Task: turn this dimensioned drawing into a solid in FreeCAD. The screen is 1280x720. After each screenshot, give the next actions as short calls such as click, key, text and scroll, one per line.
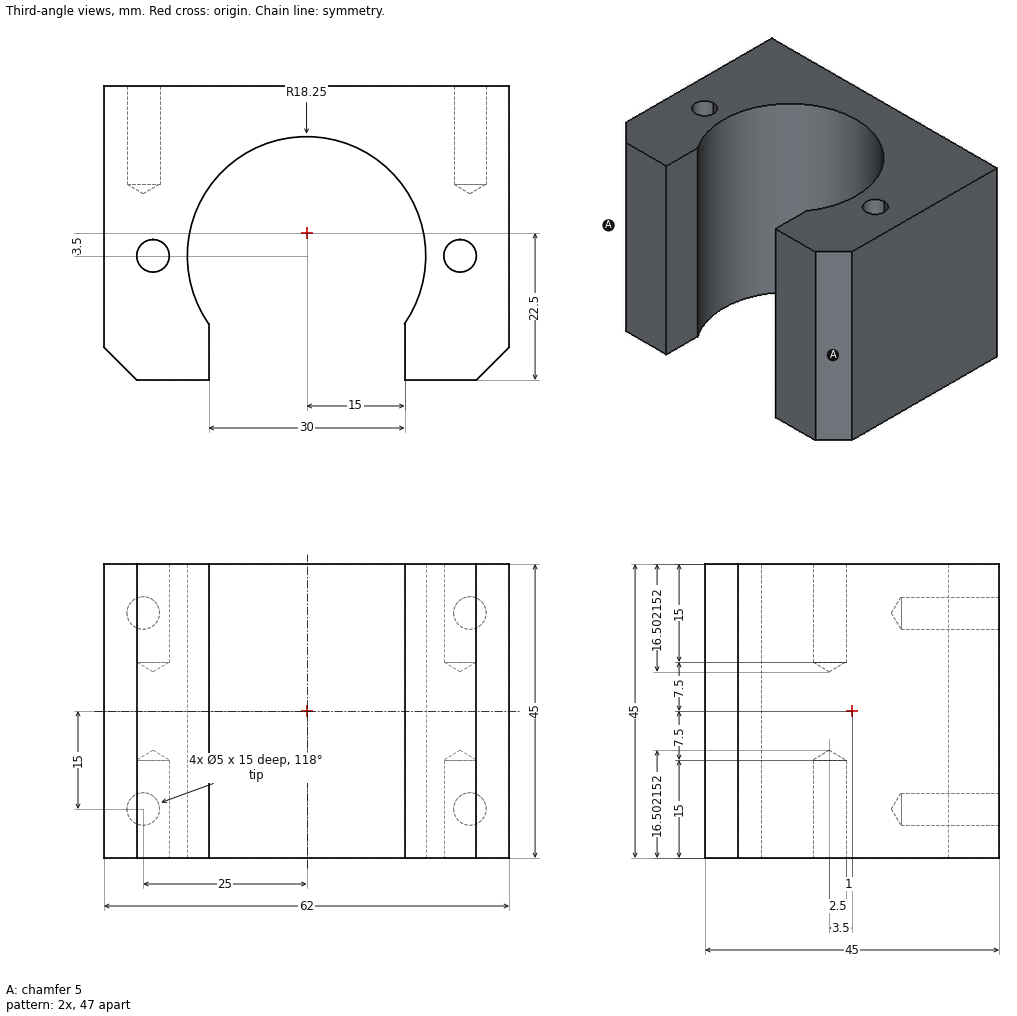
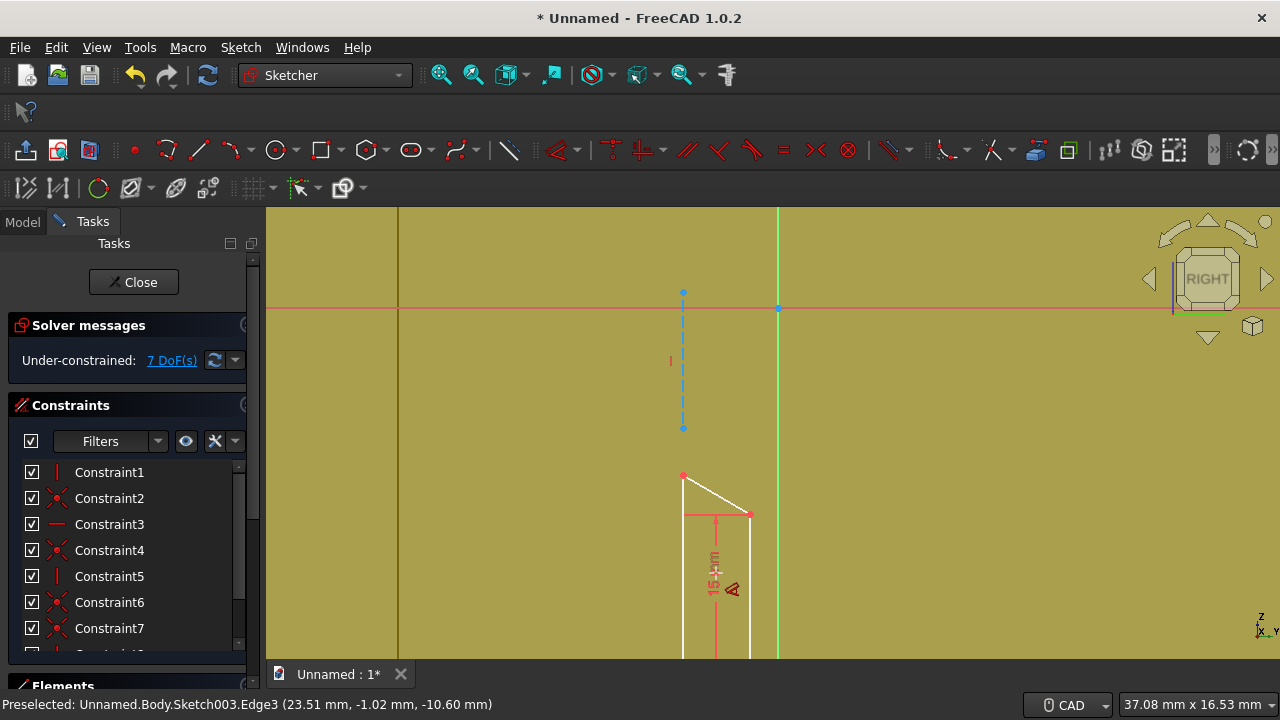
scroll(683, 291, down, 4)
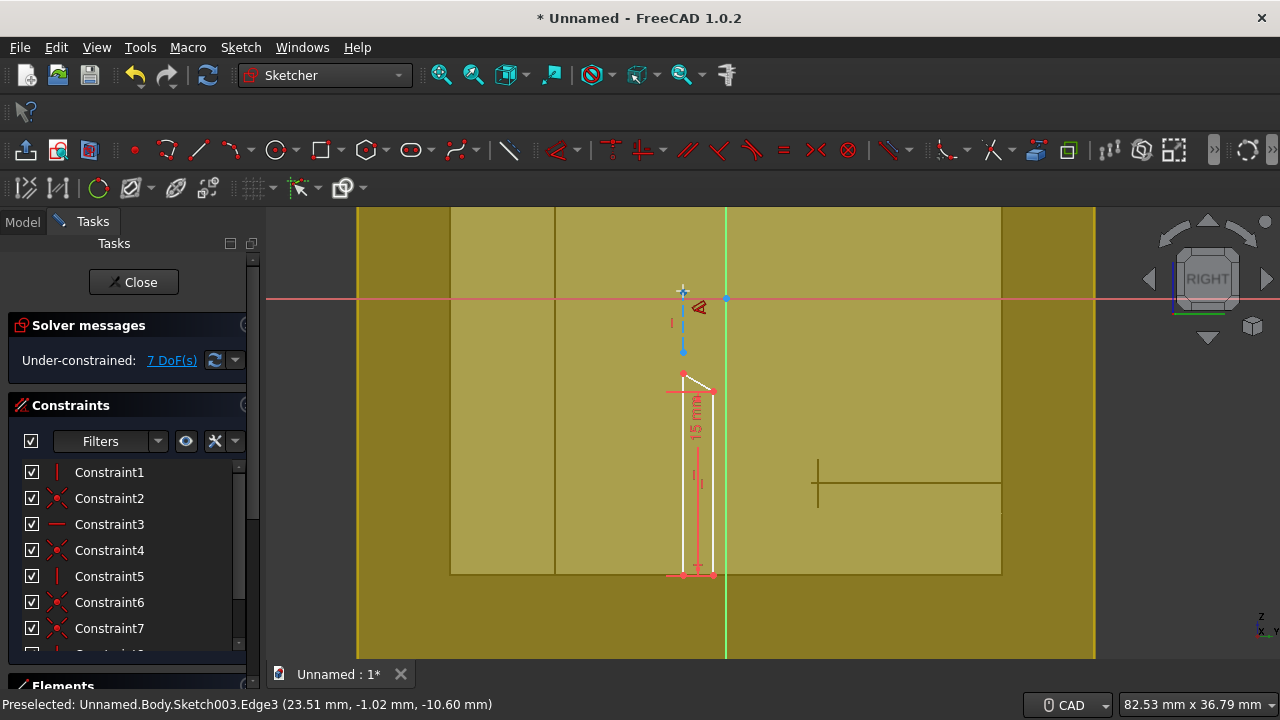
scroll(713, 576, up, 6)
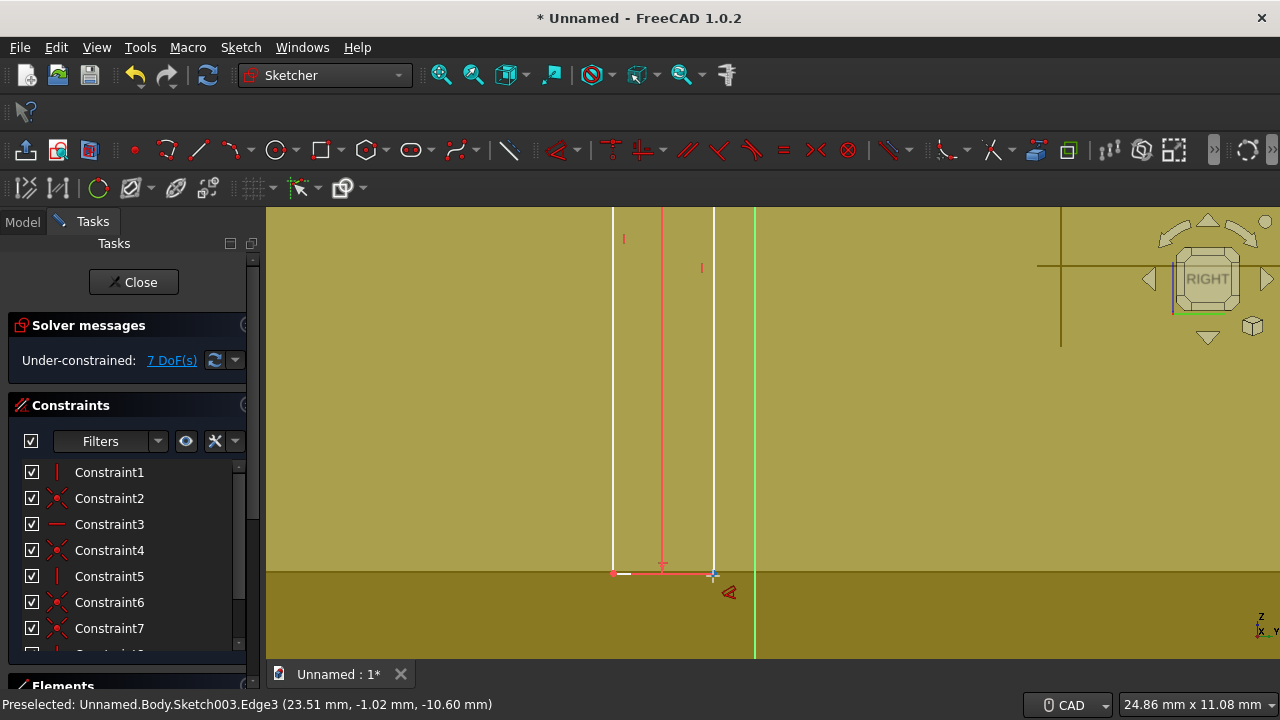
click(714, 574)
click(734, 608)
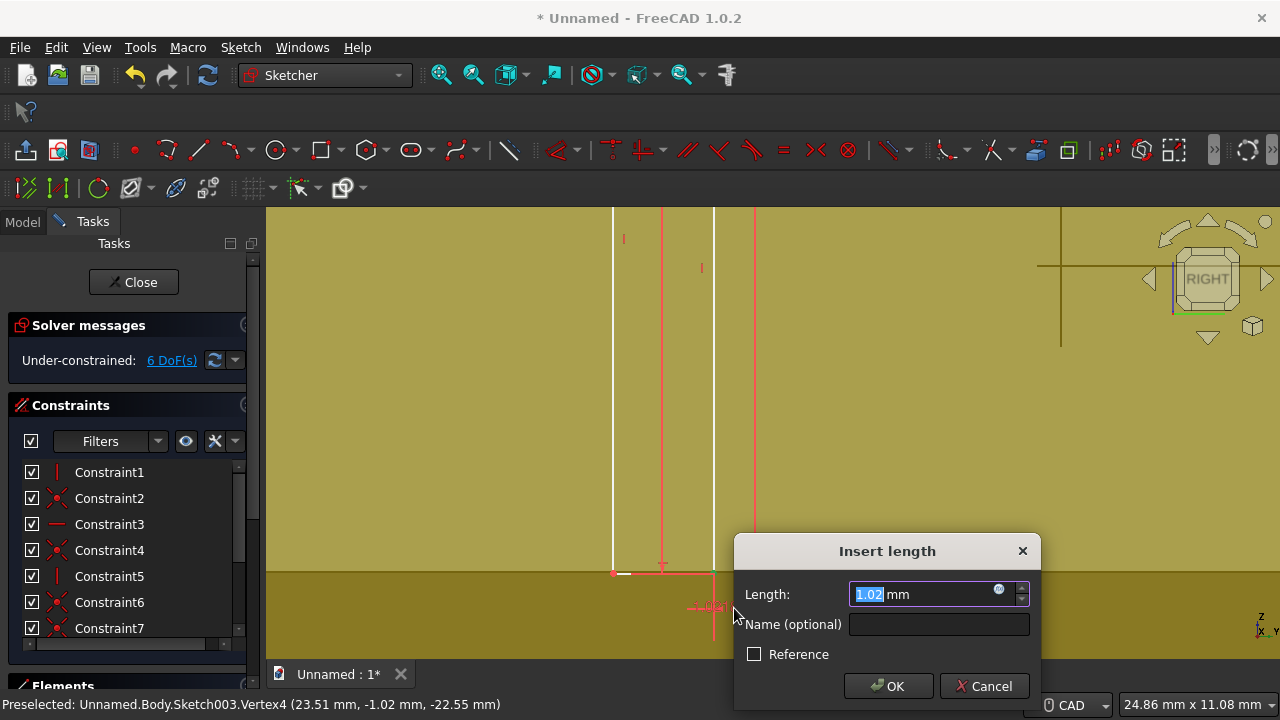
text(1)
key(Return)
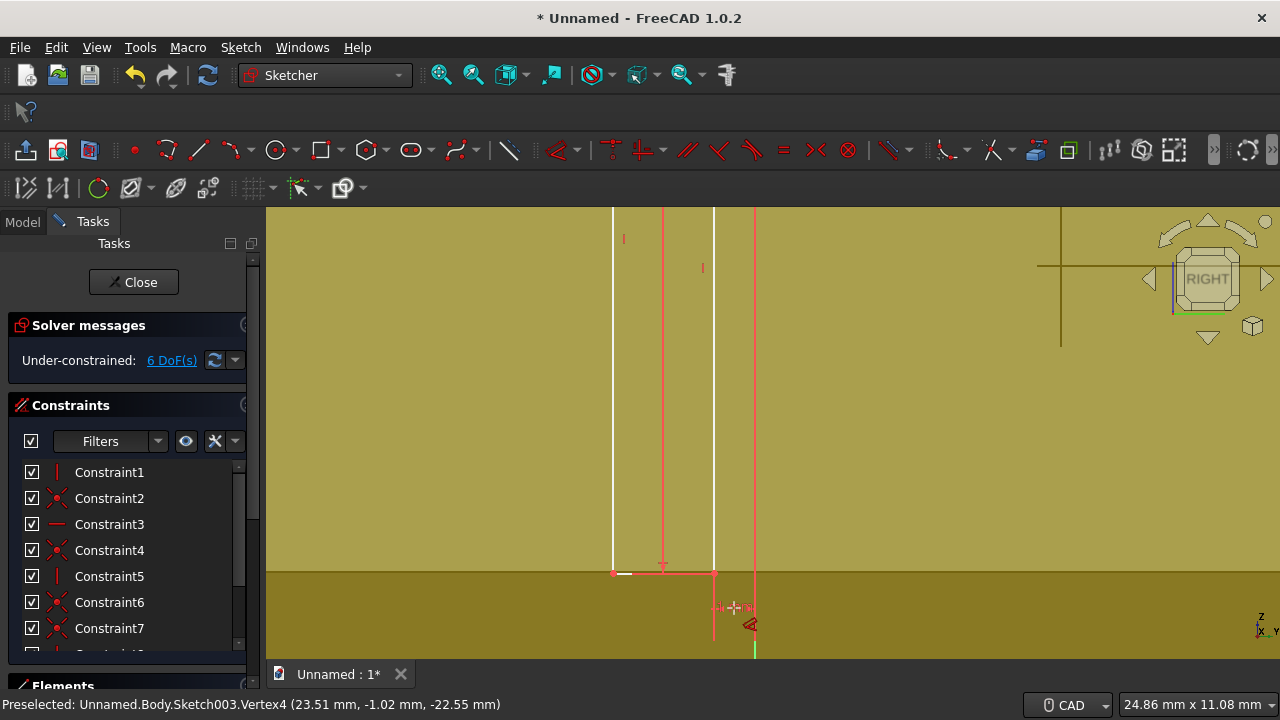
click(644, 574)
click(664, 608)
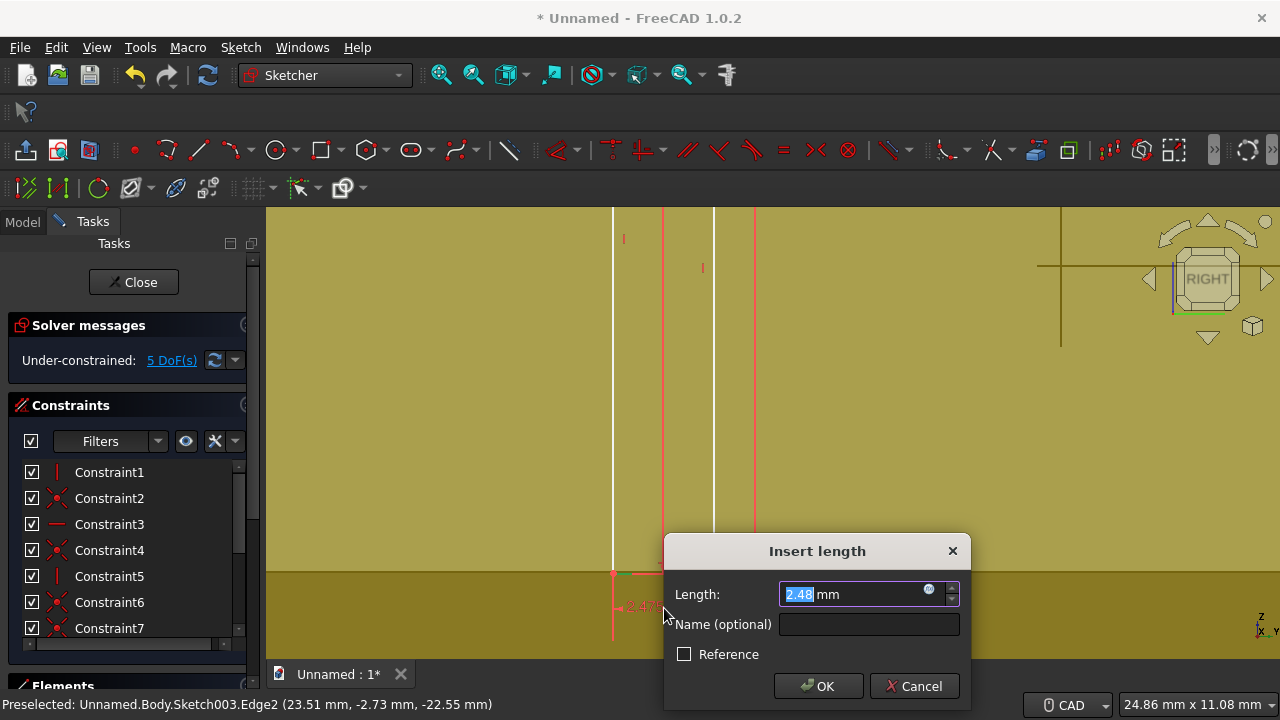
text(2.5)
key(Return)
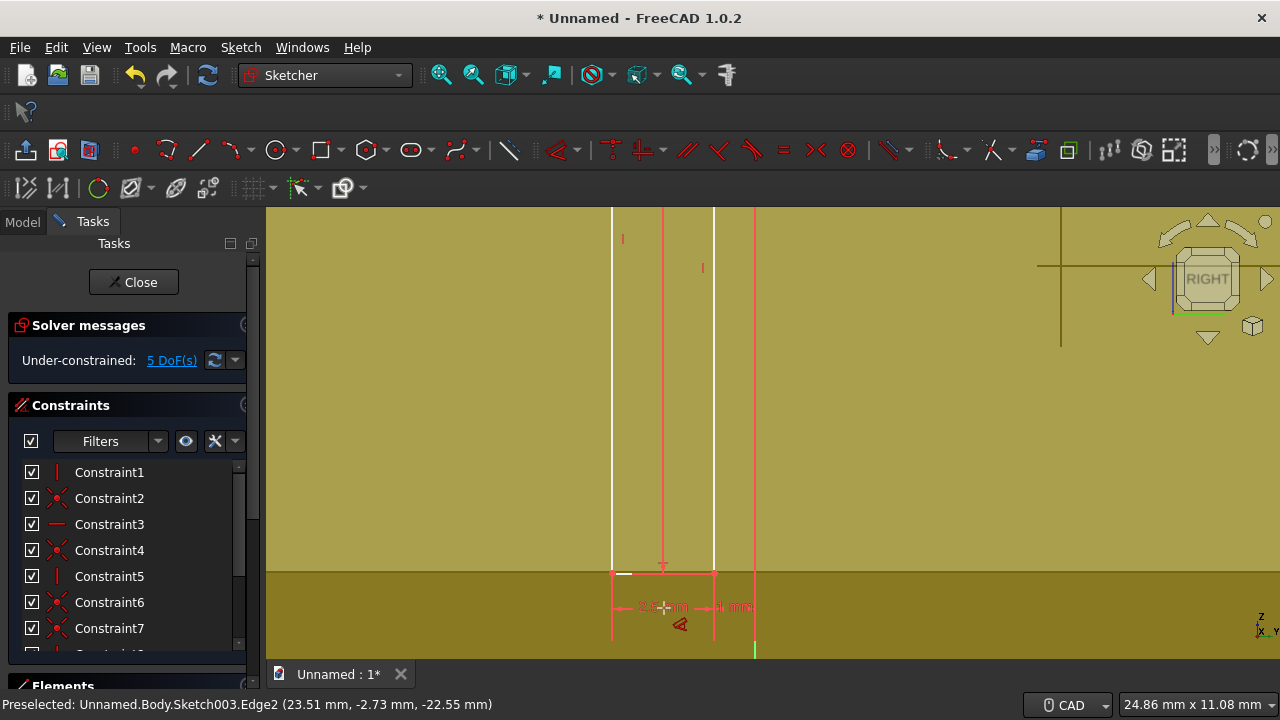
scroll(713, 576, down, 6)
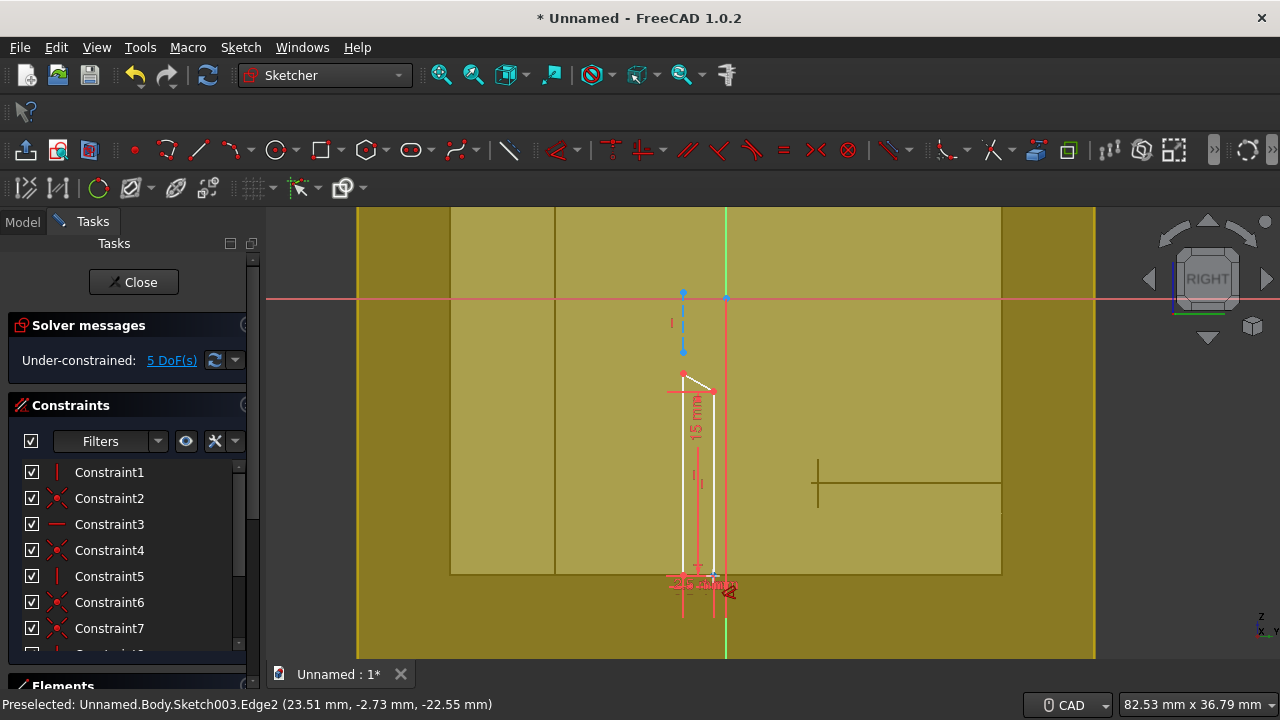
click(714, 392)
click(760, 345)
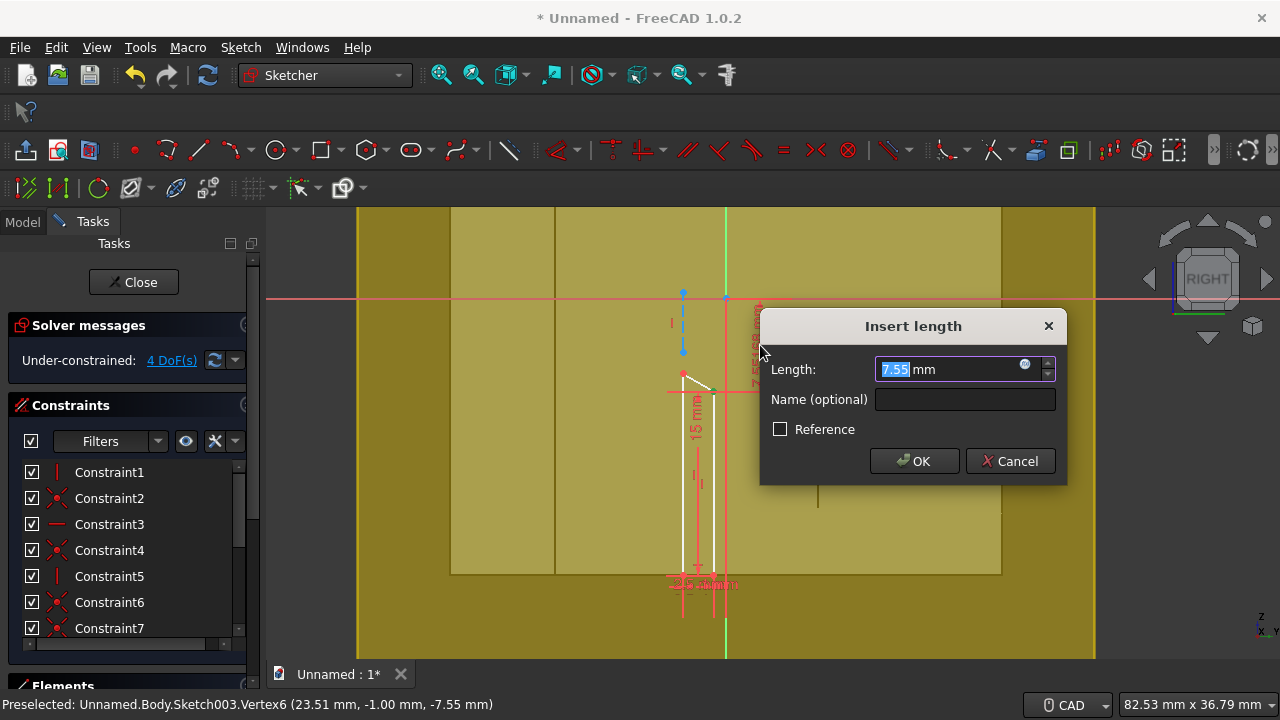
text(7.5)
key(Return)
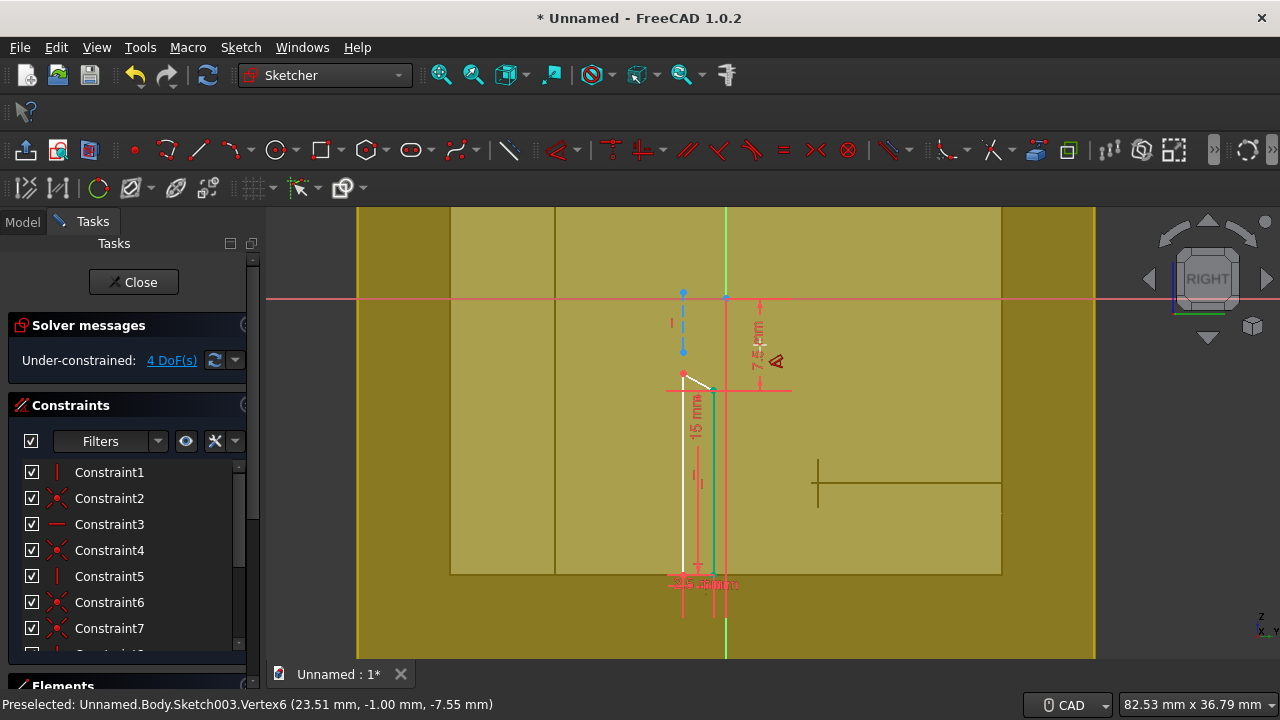
click(683, 353)
click(705, 265)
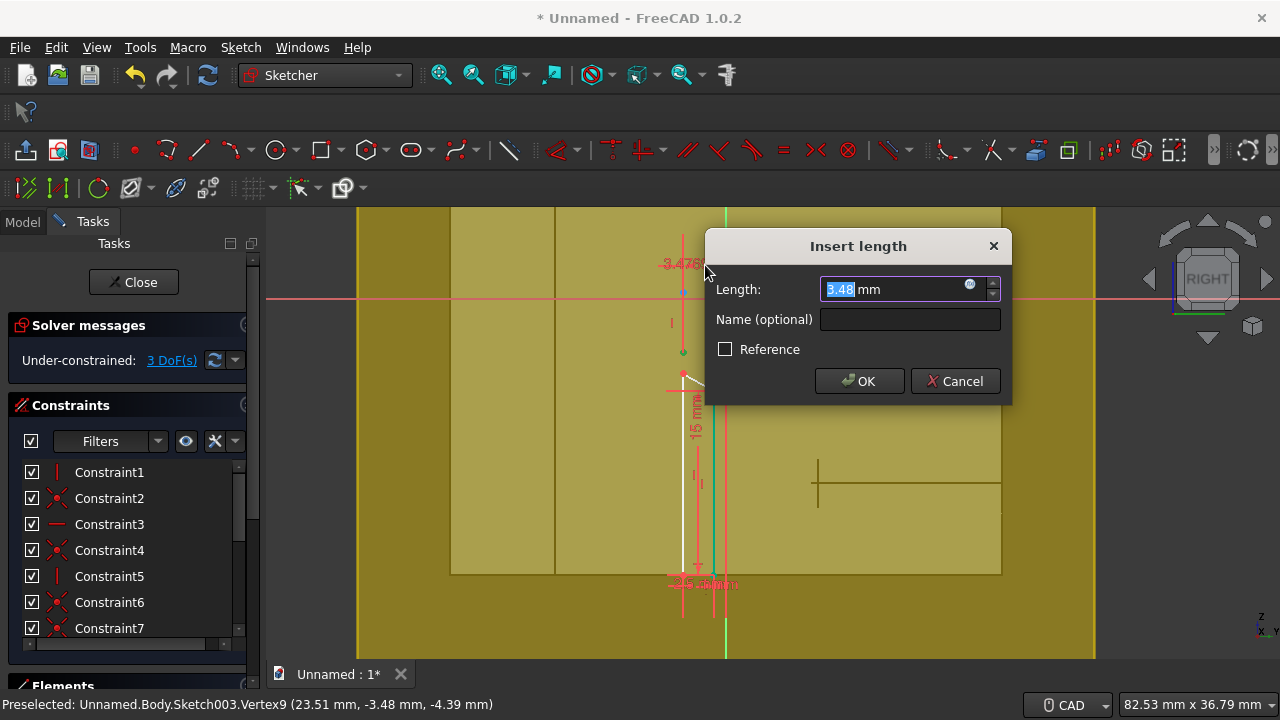
text(3.5)
key(Return)